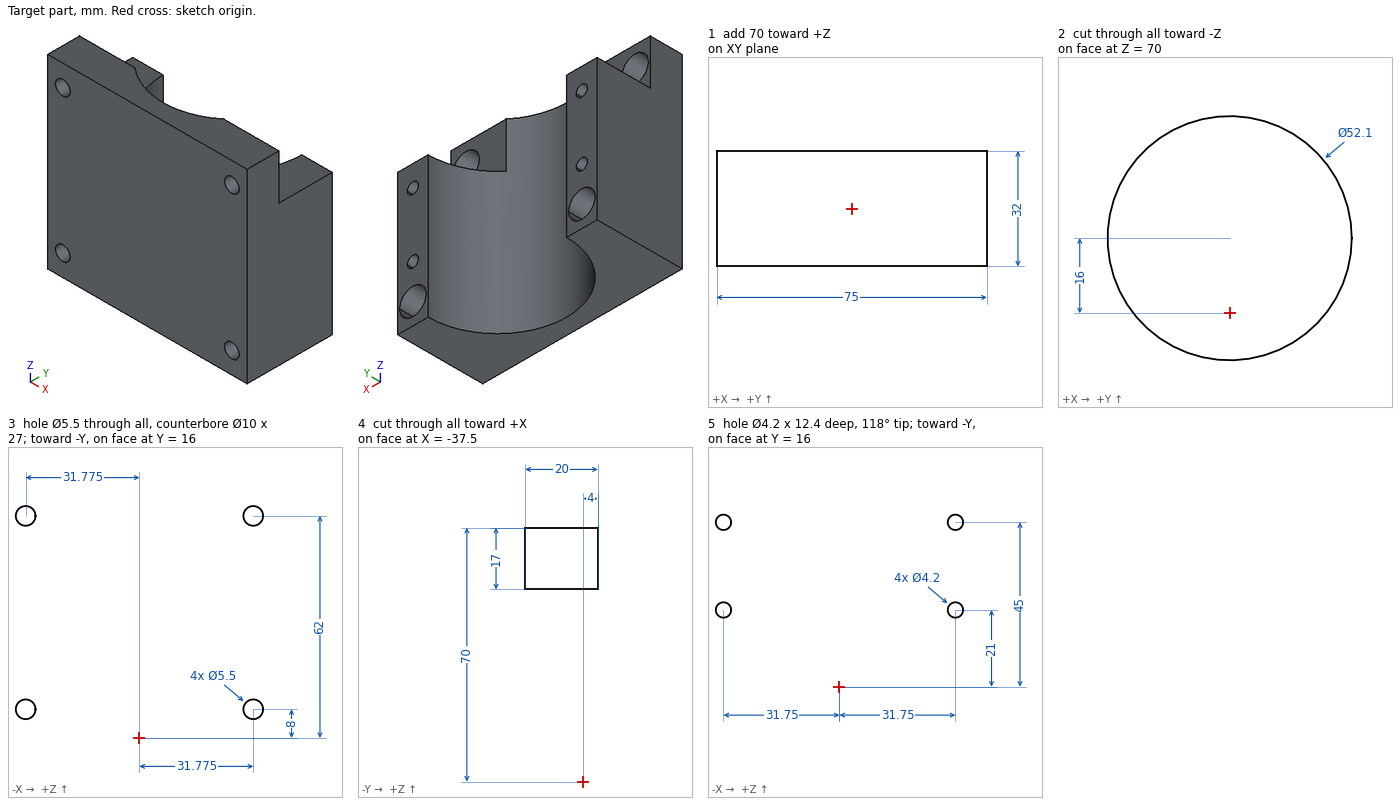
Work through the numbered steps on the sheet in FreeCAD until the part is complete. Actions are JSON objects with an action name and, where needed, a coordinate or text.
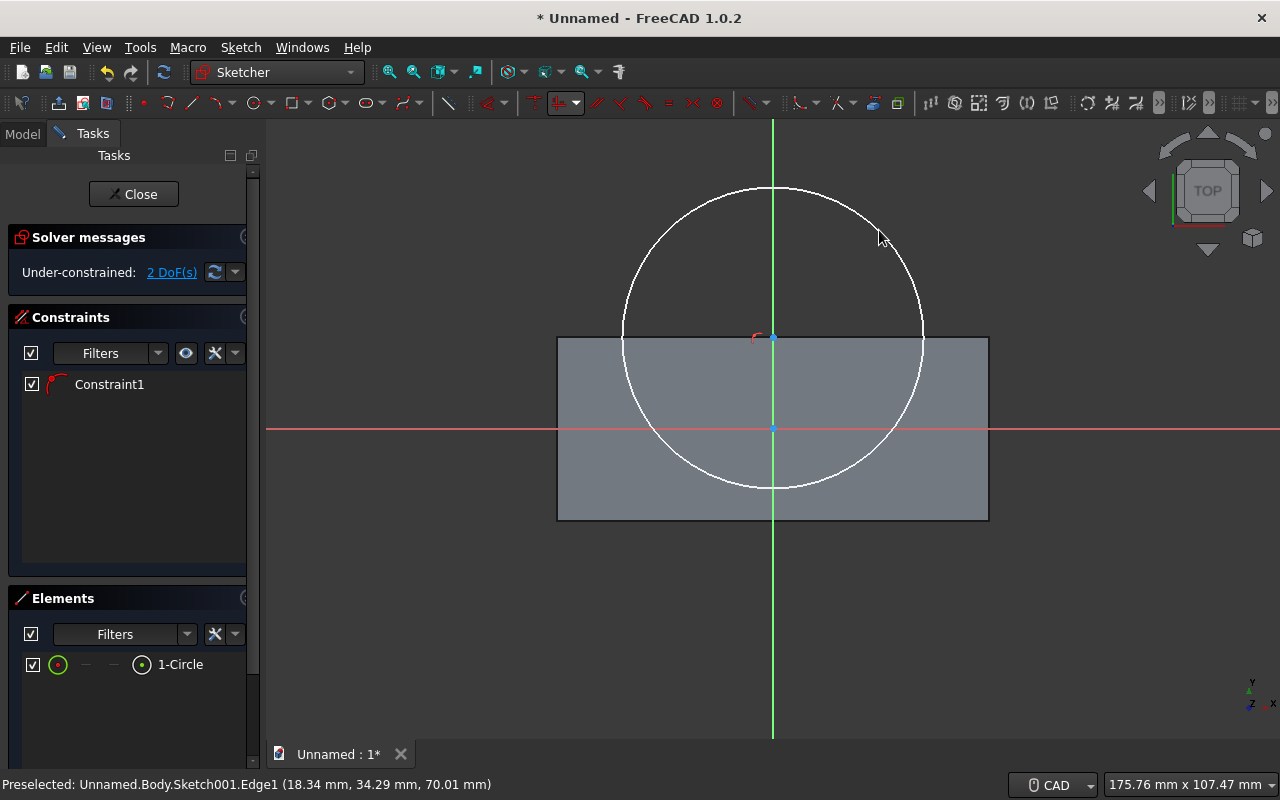
{"action": "left_click", "coordinate": [488, 104]}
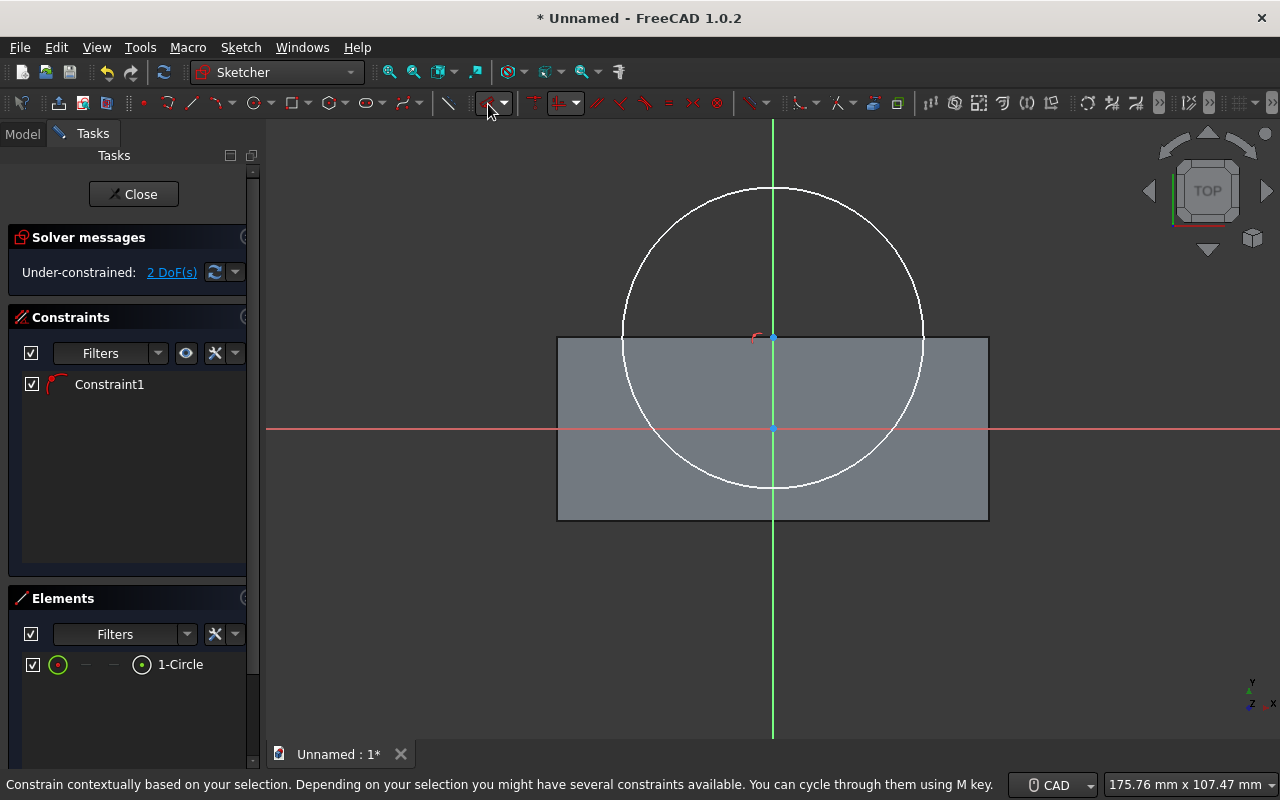
{"action": "left_click", "coordinate": [879, 231]}
{"action": "left_click", "coordinate": [902, 208]}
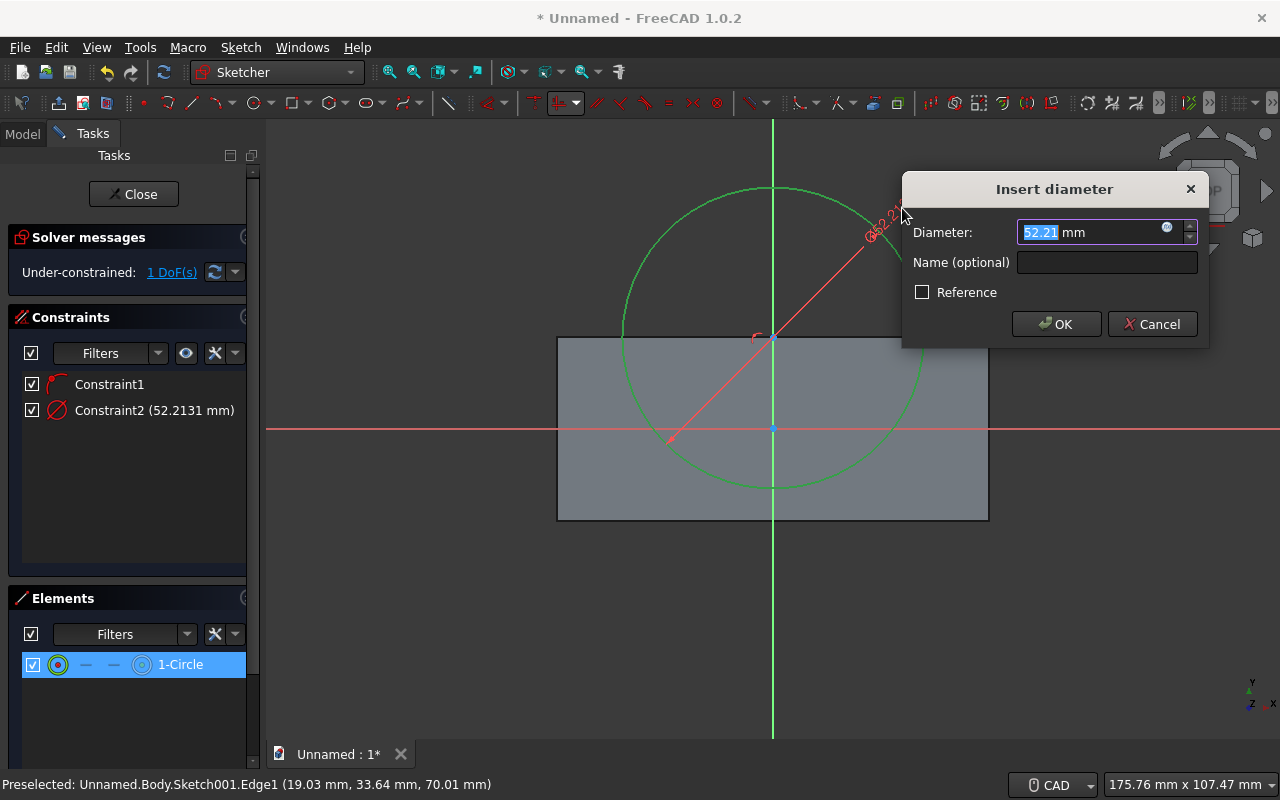
{"action": "type", "text": "52.1"}
{"action": "key", "text": "Return"}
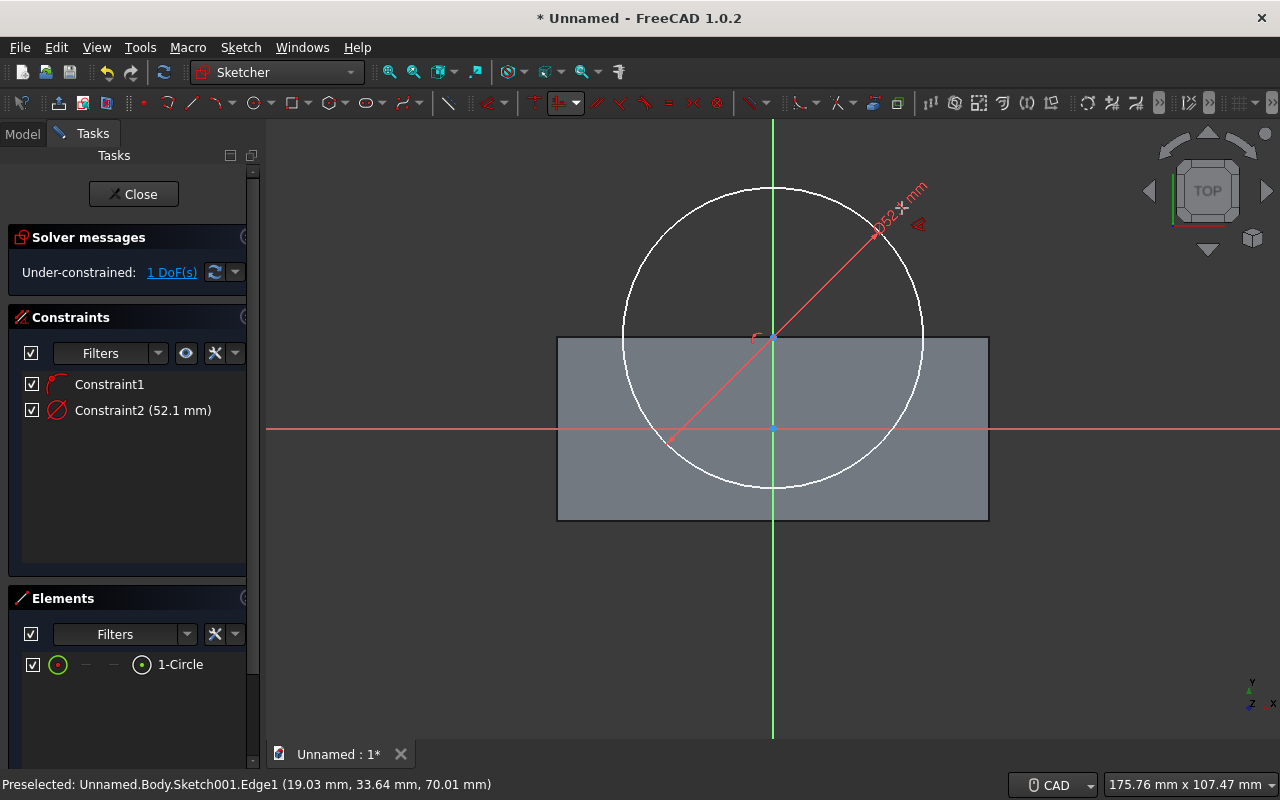
{"action": "left_click", "coordinate": [773, 338]}
{"action": "left_click", "coordinate": [807, 384]}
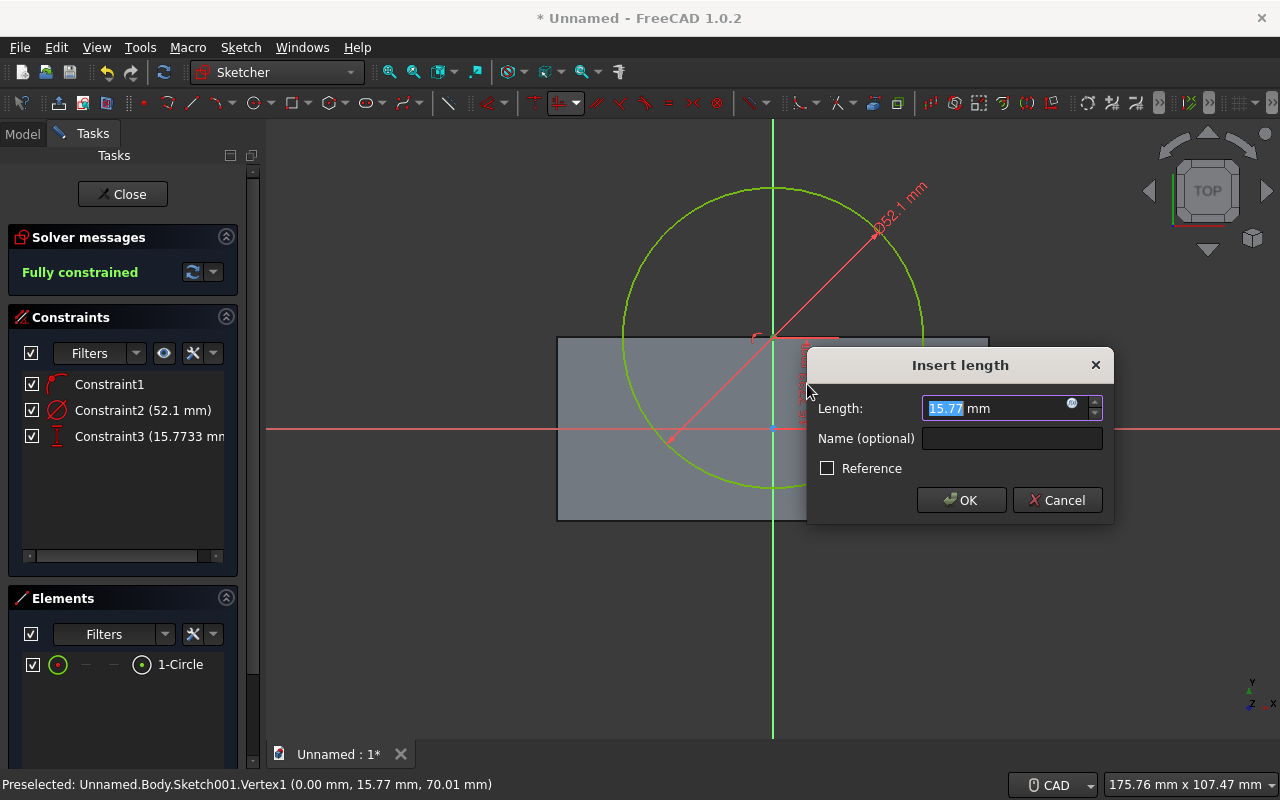
{"action": "type", "text": "16"}
{"action": "key", "text": "Return"}
{"action": "key", "text": "Escape"}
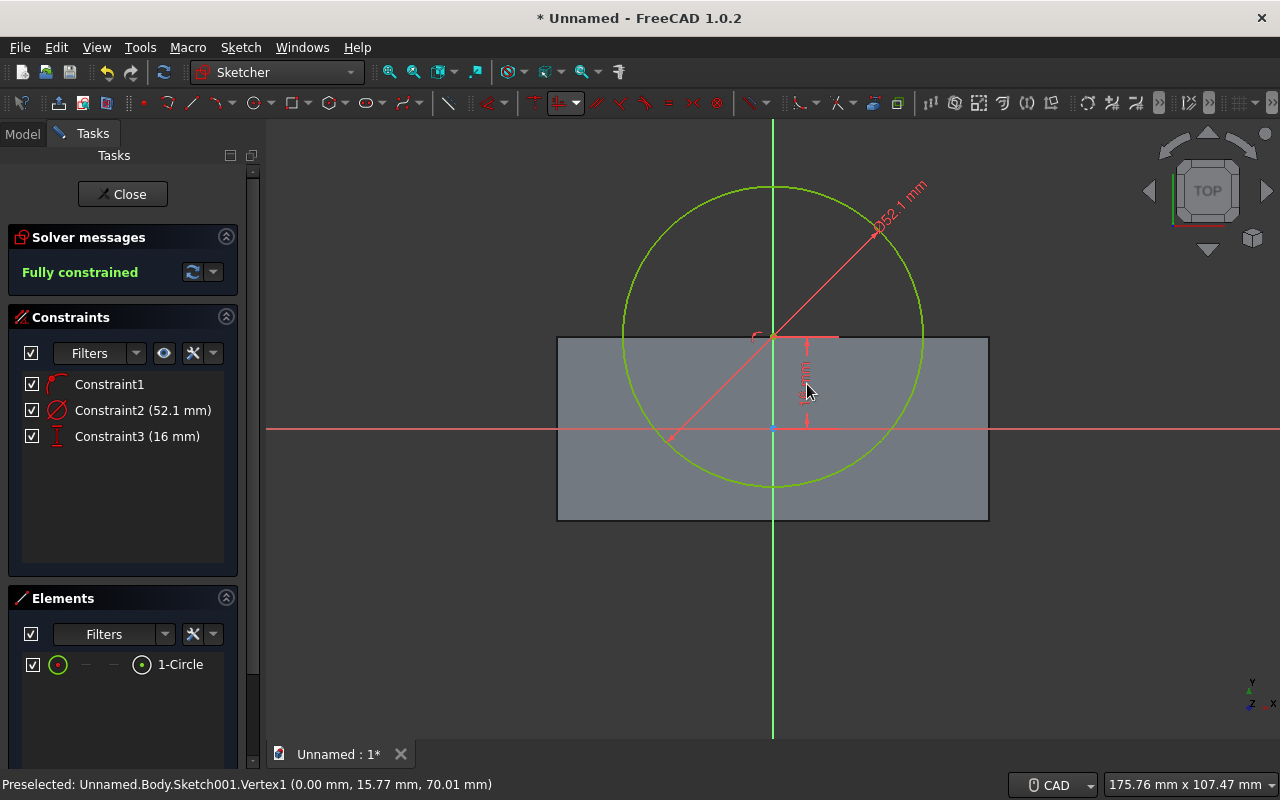
{"action": "left_click", "coordinate": [123, 194]}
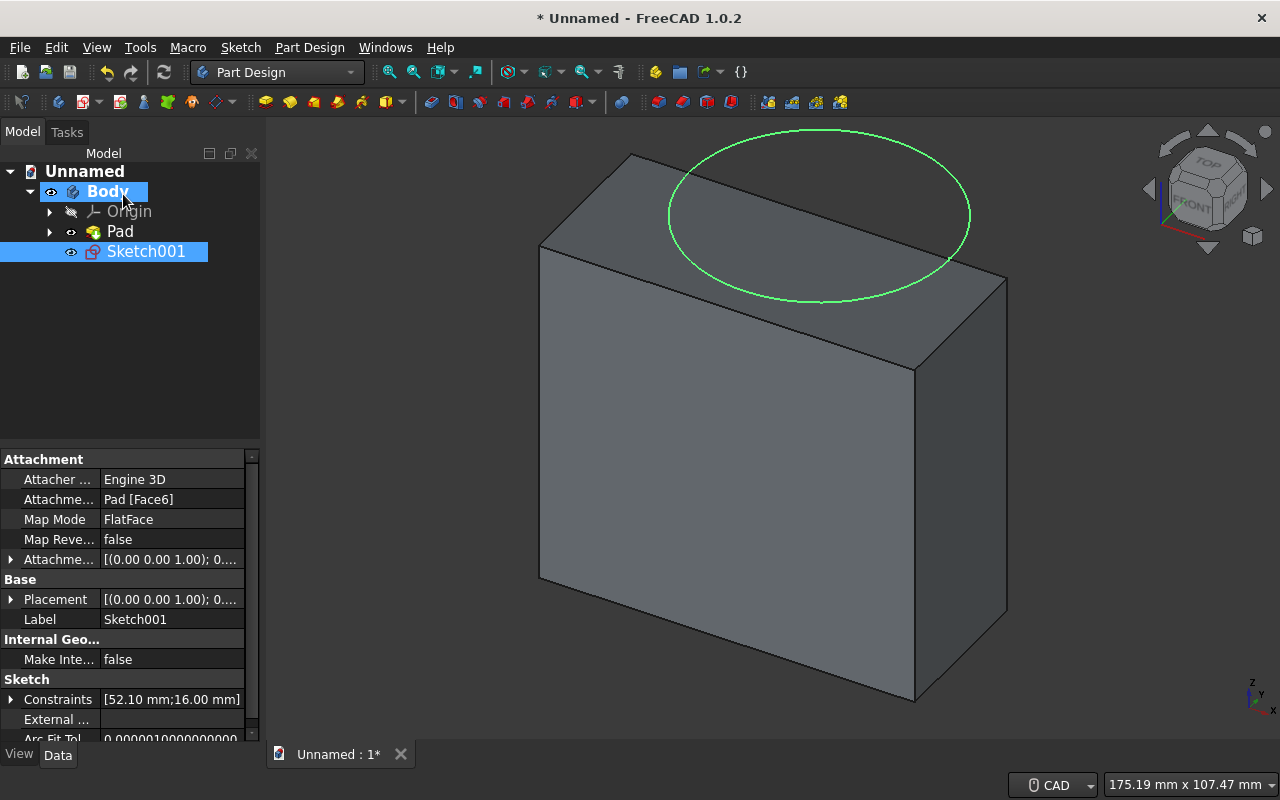
{"action": "left_click", "coordinate": [432, 102]}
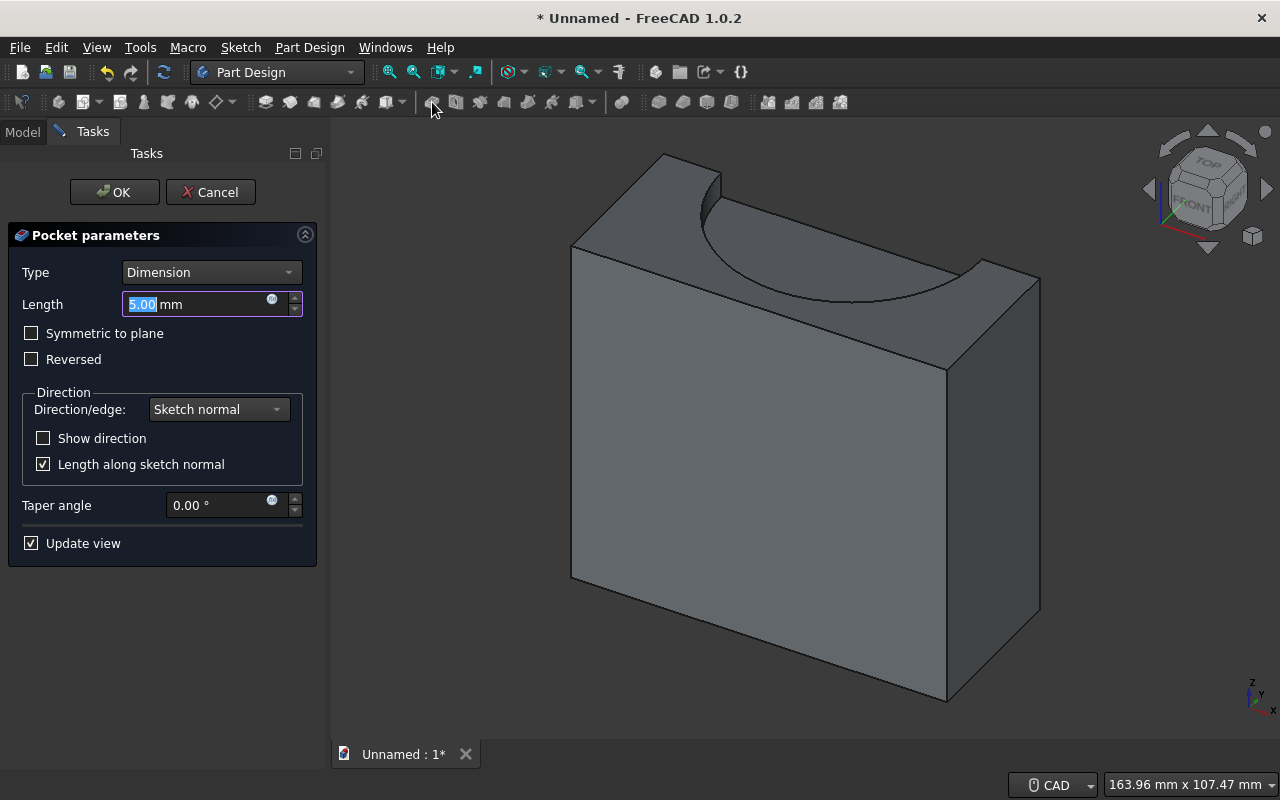
{"action": "left_click", "coordinate": [212, 272]}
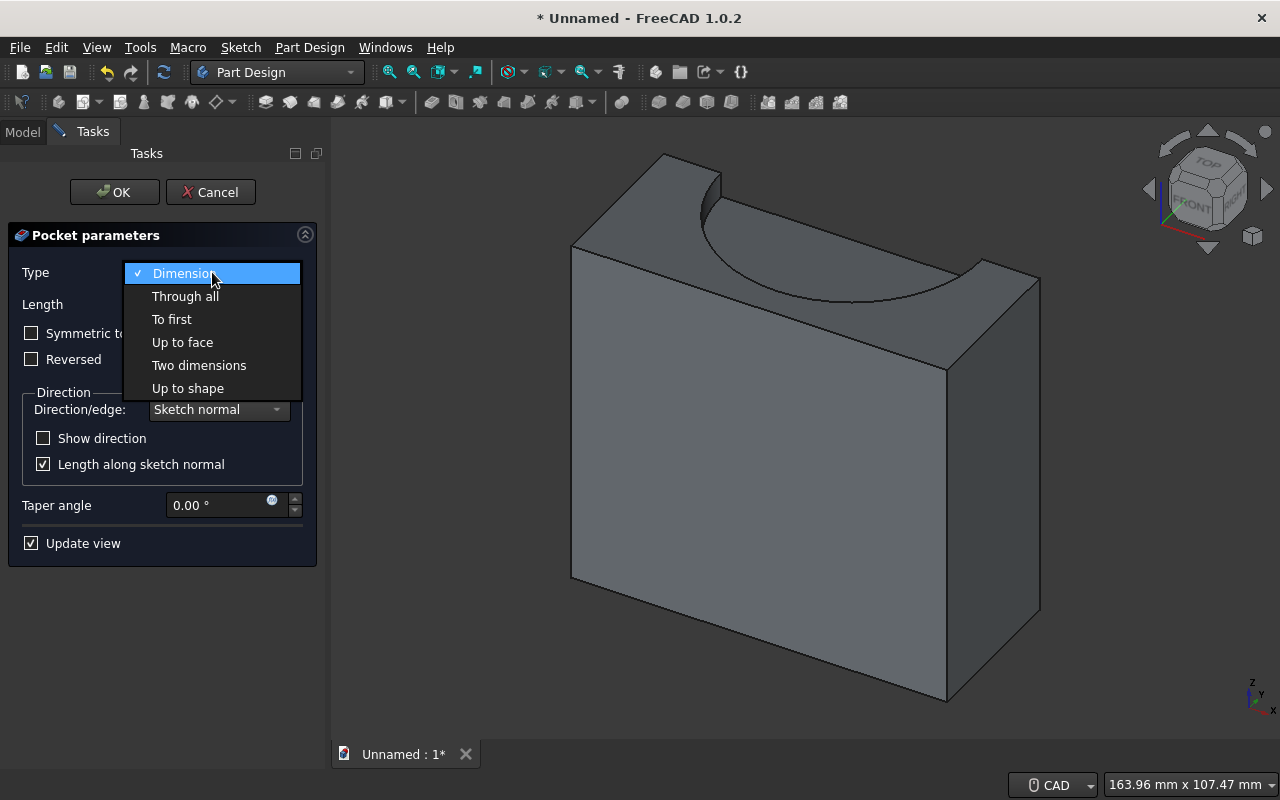
{"action": "left_click", "coordinate": [212, 296]}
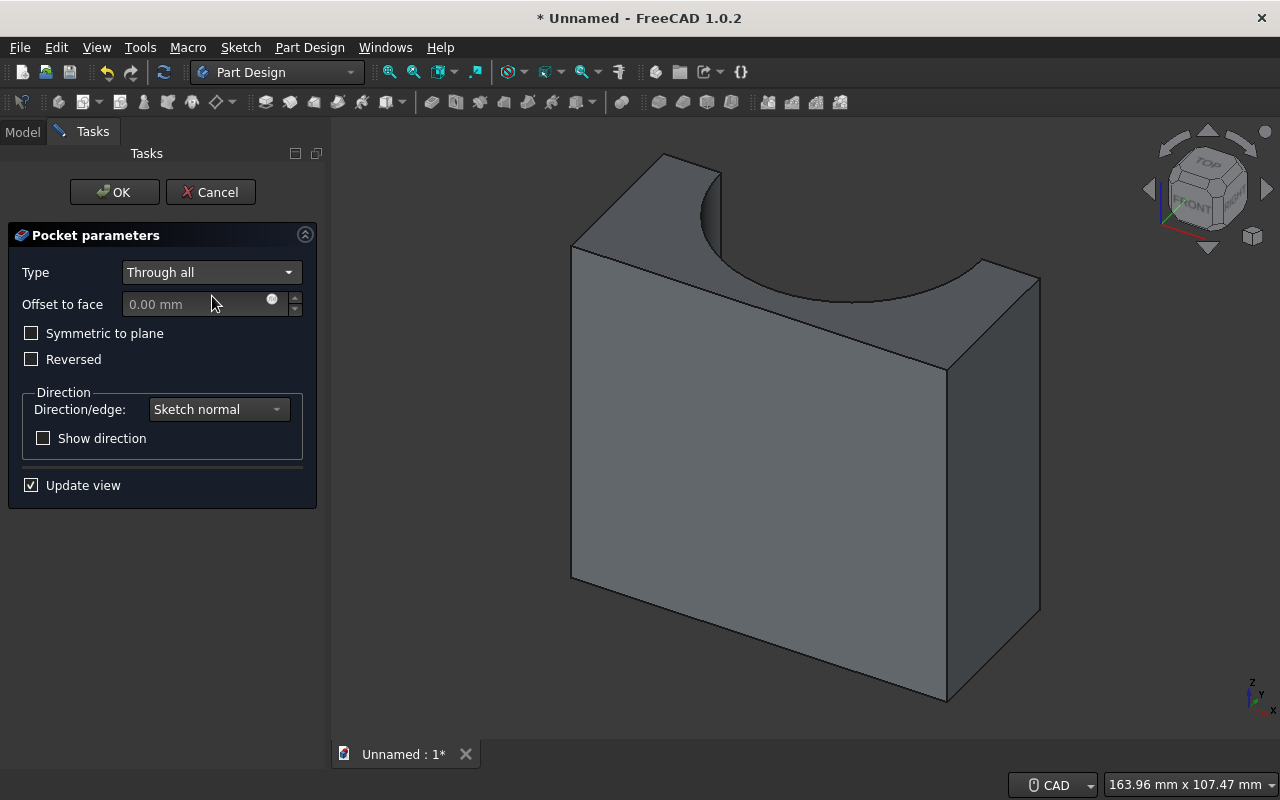
{"action": "left_click", "coordinate": [115, 192]}